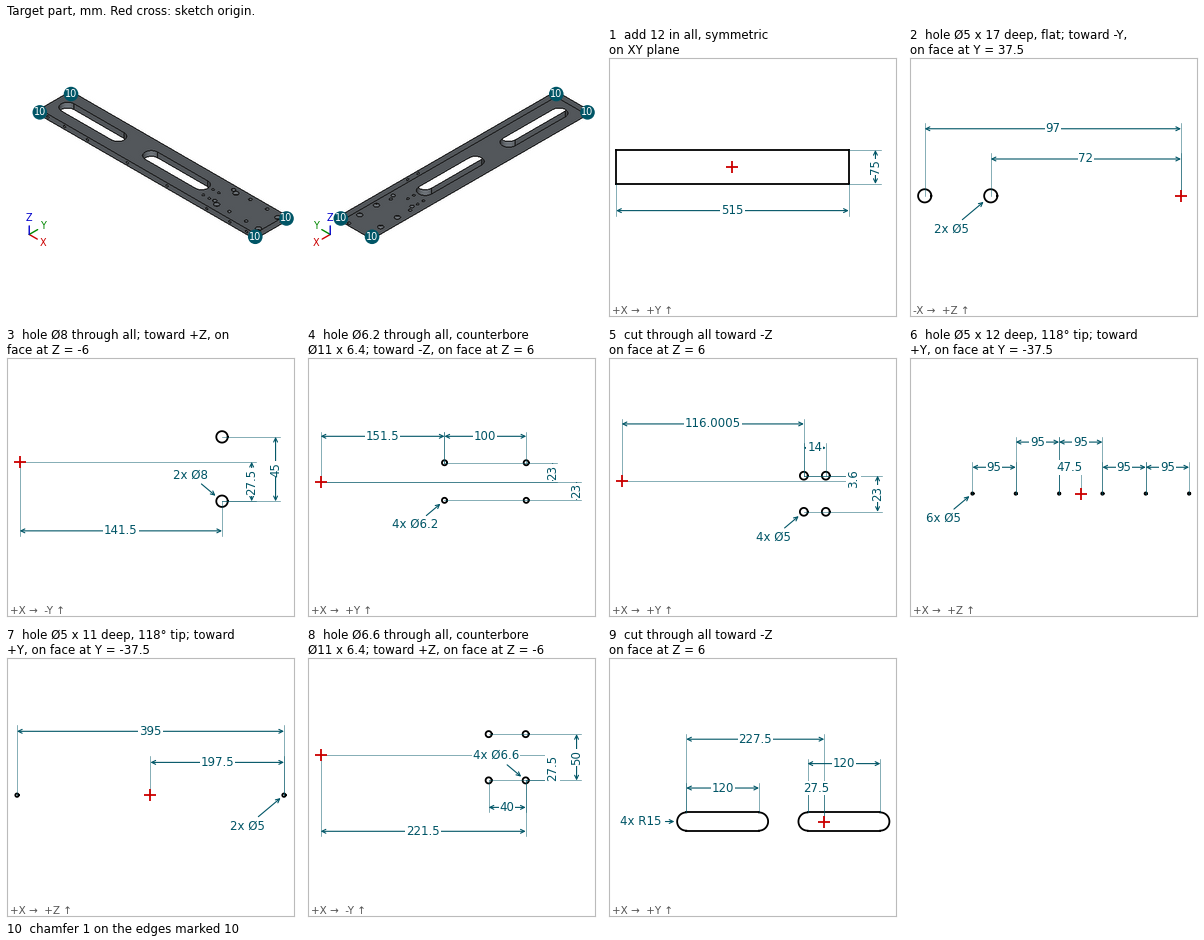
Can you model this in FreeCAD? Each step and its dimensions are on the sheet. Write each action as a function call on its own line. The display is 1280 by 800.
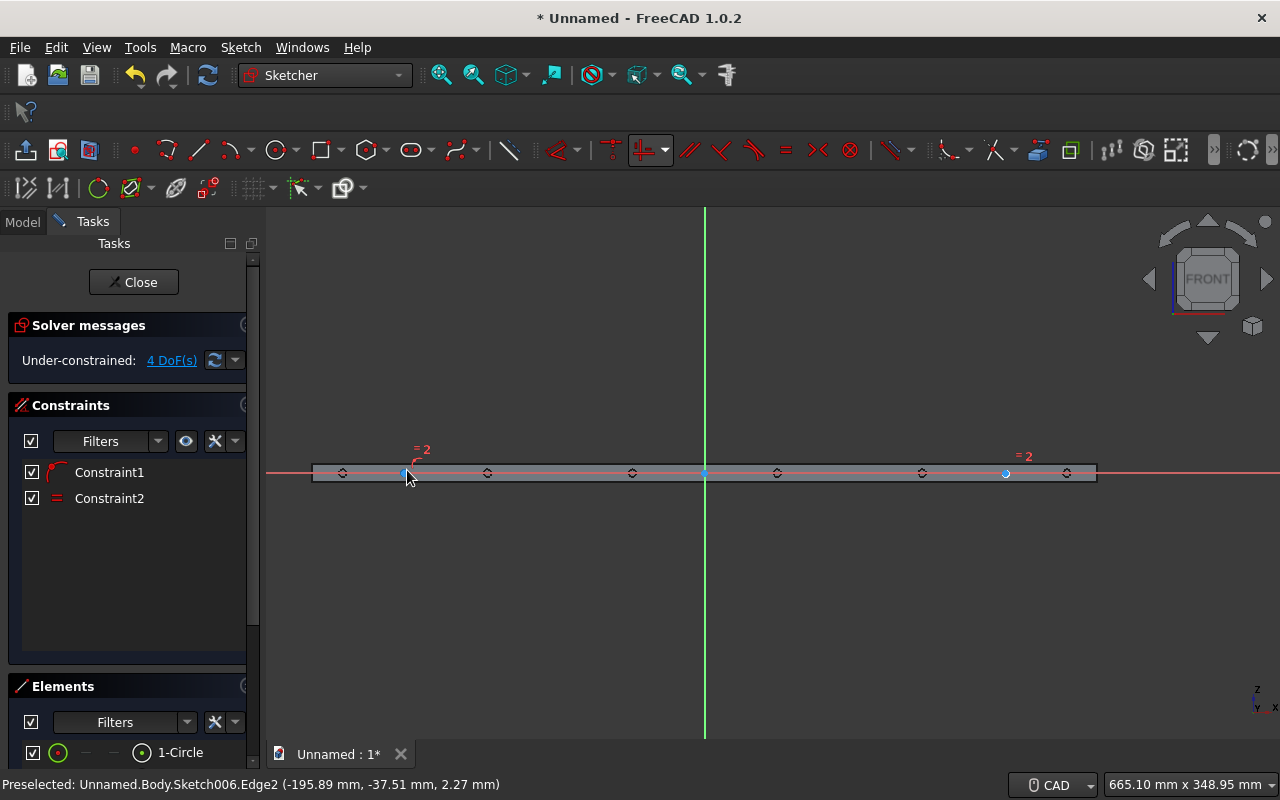
click(1006, 474)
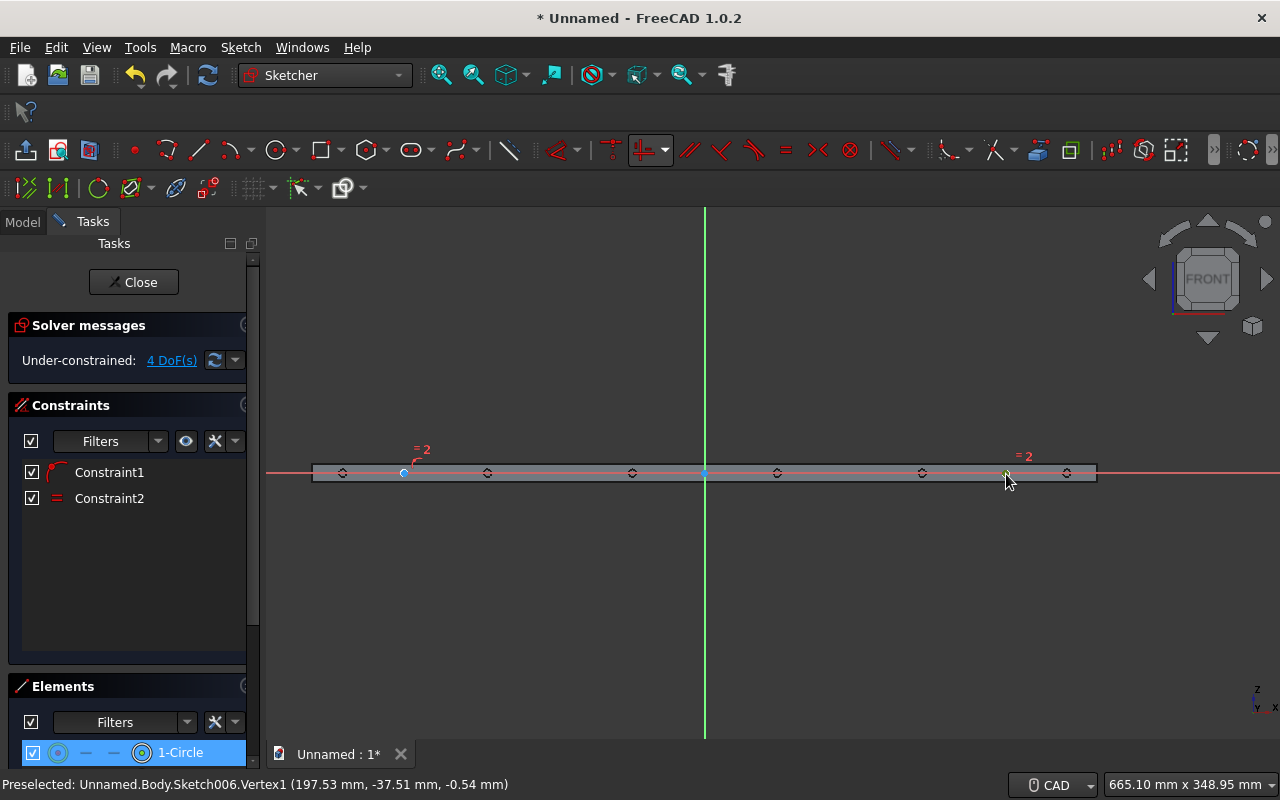
click(353, 473)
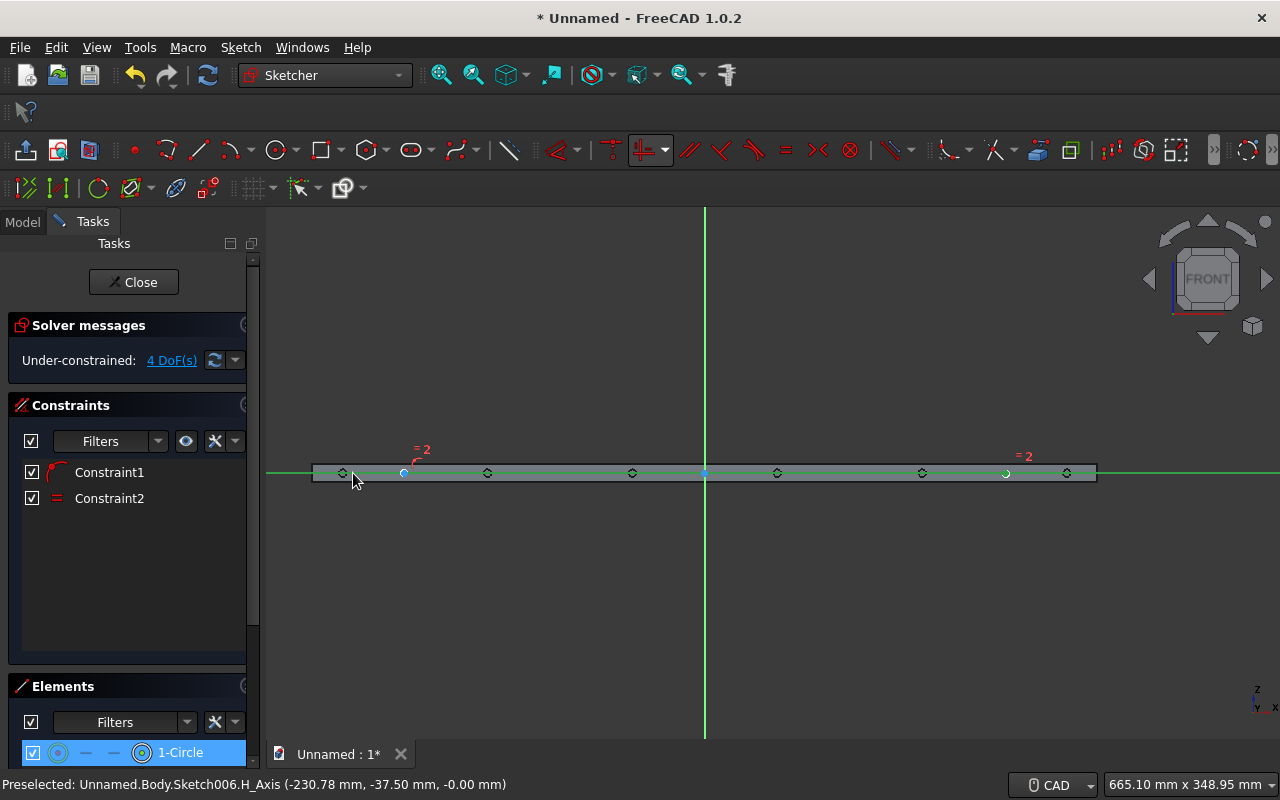
click(612, 150)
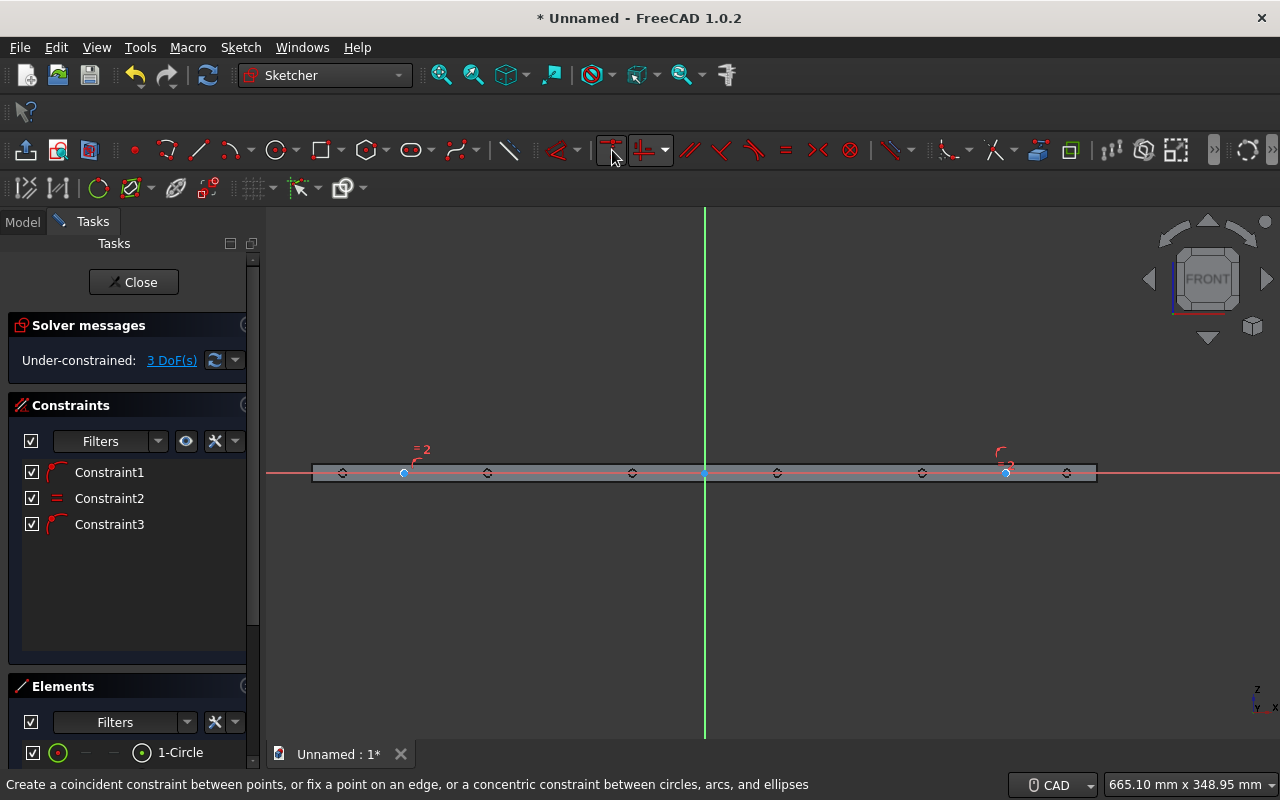
key(d)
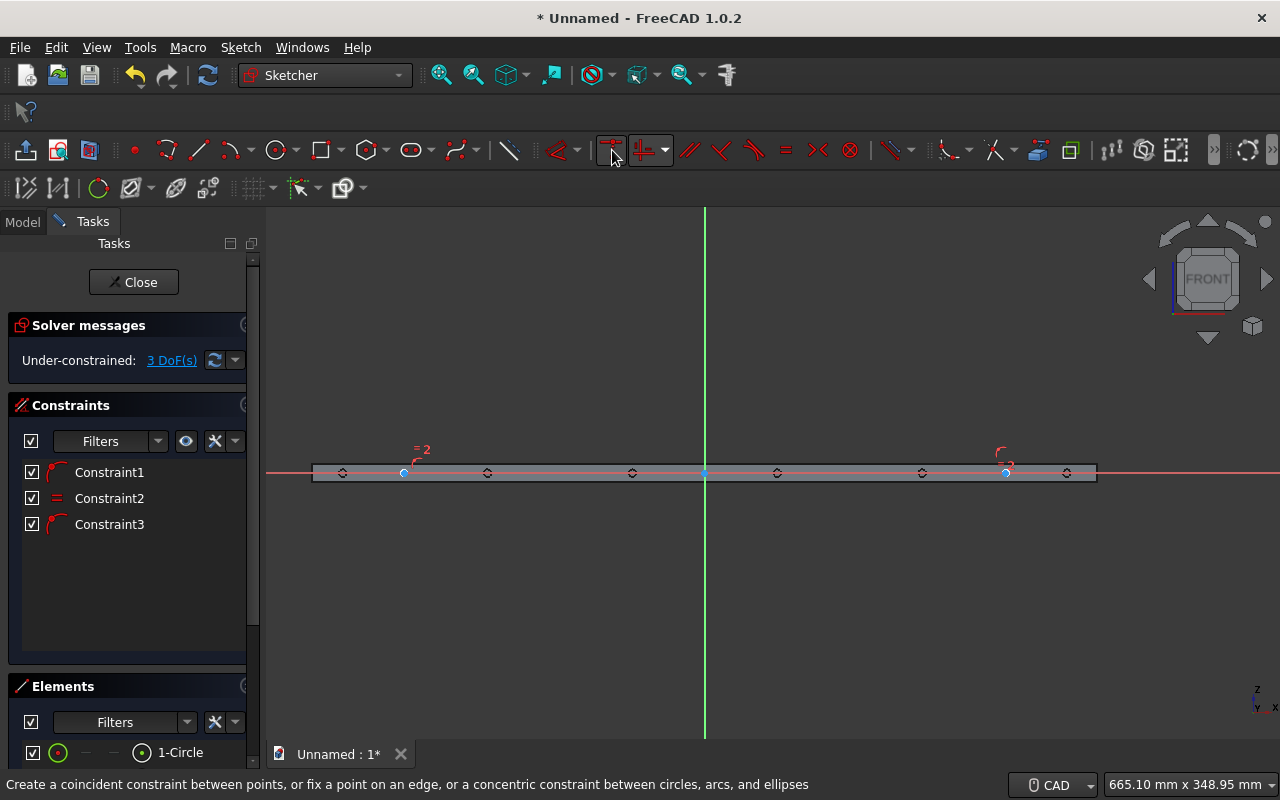
scroll(1008, 476, up, 9)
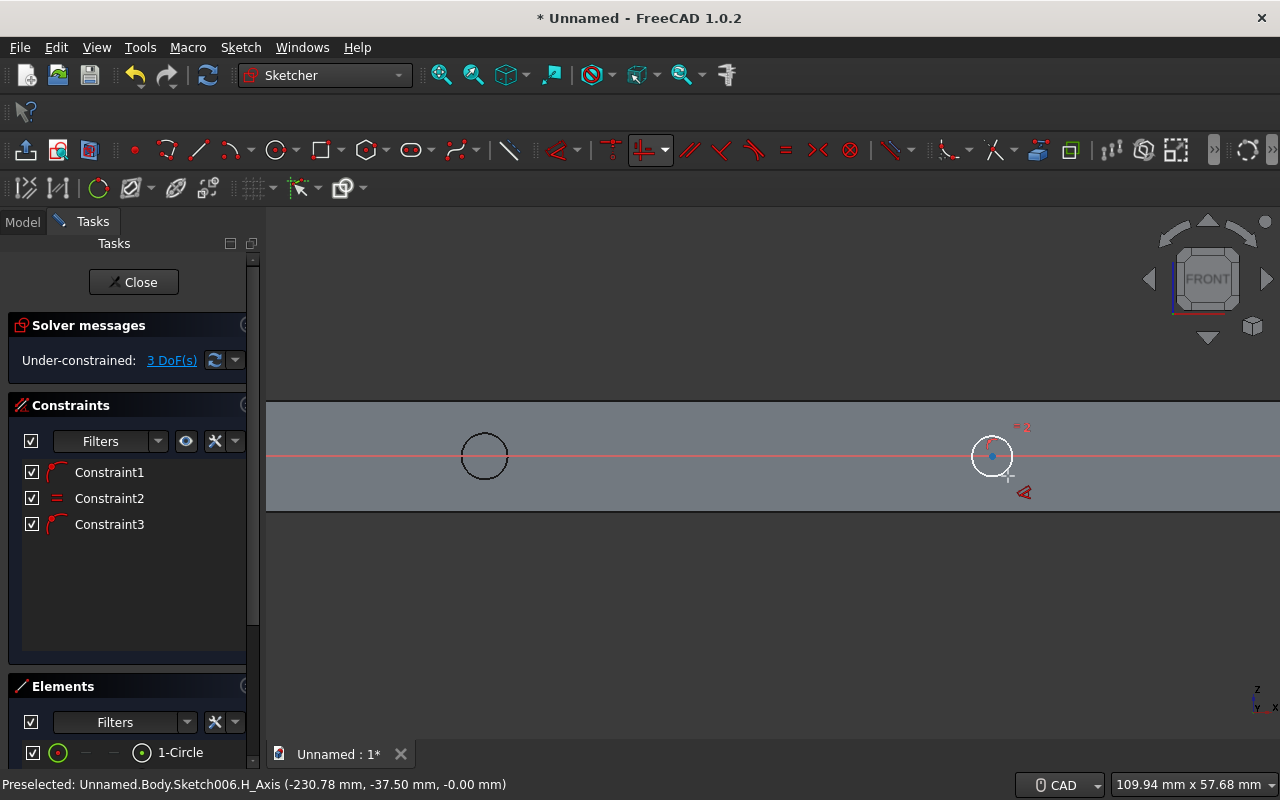
click(1006, 471)
click(1028, 494)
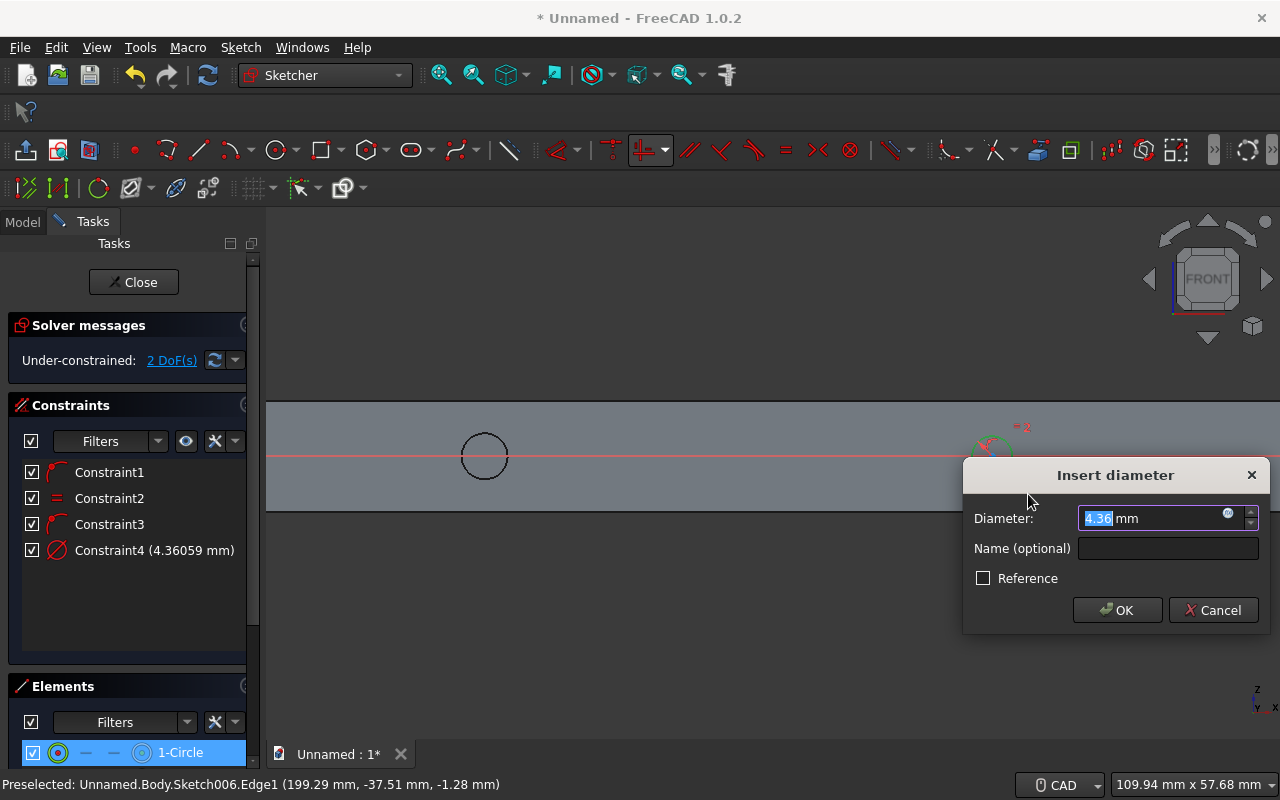
text(5)
key(Return)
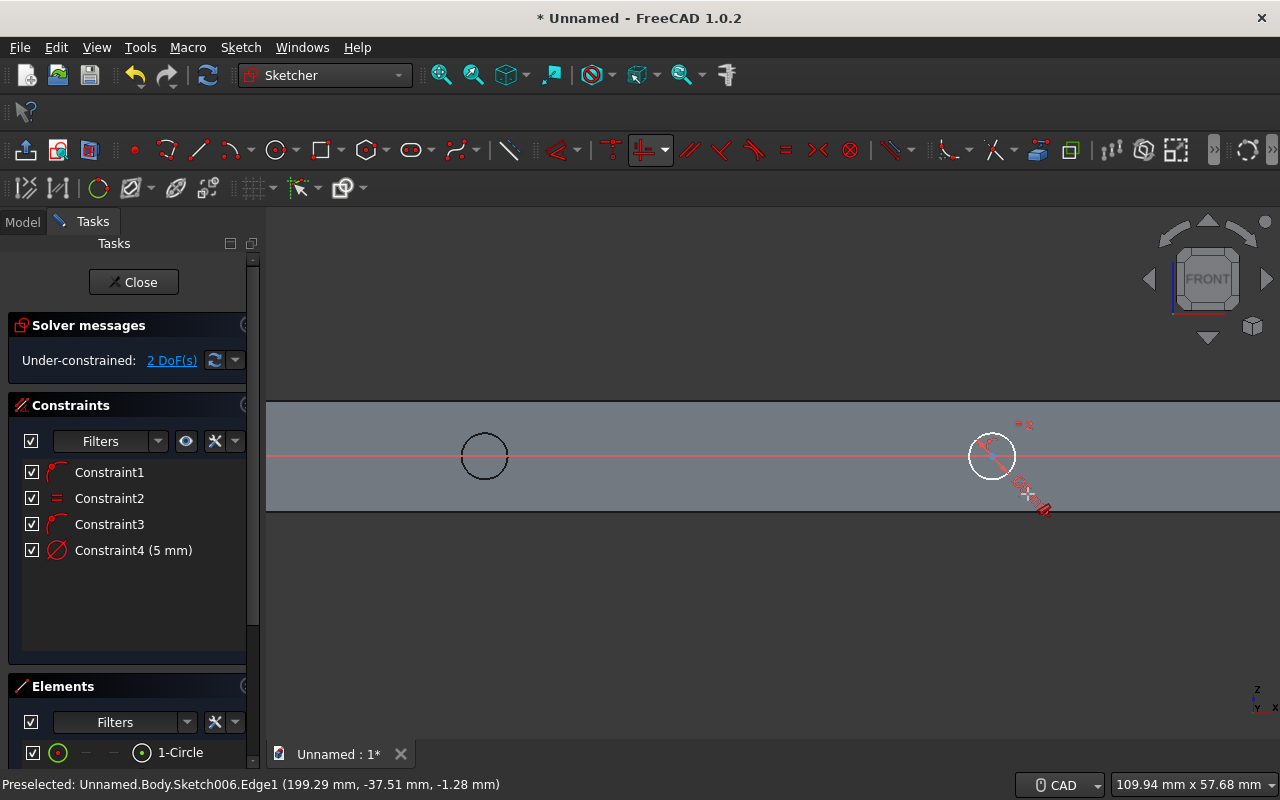
scroll(1008, 476, down, 9)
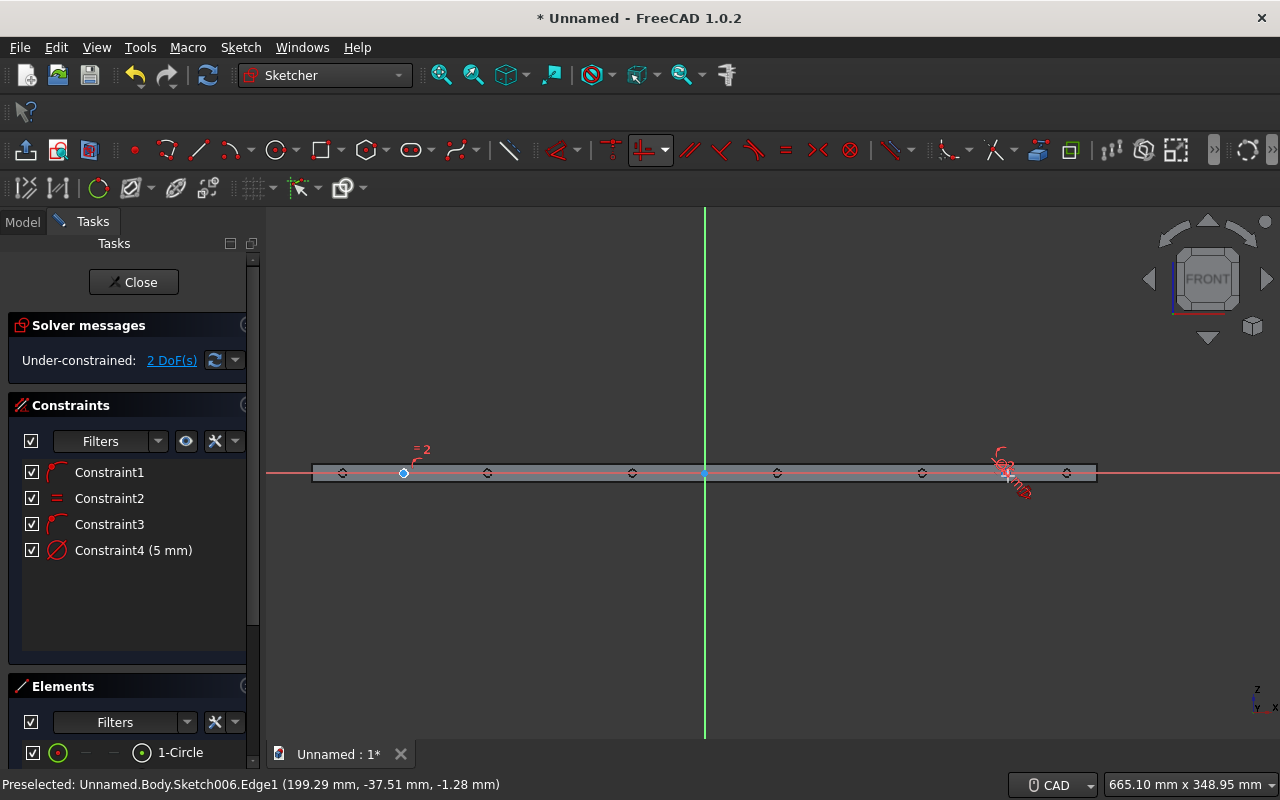
click(1006, 473)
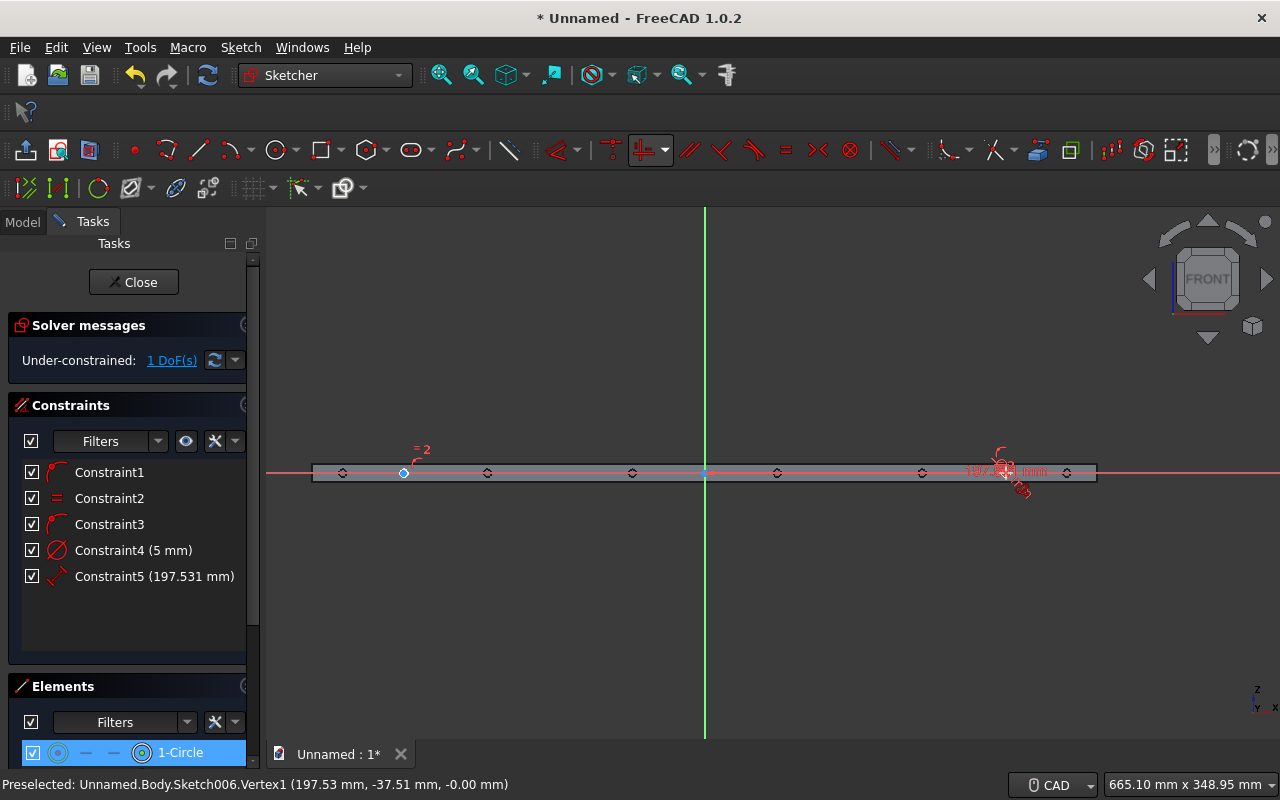
click(404, 473)
click(567, 507)